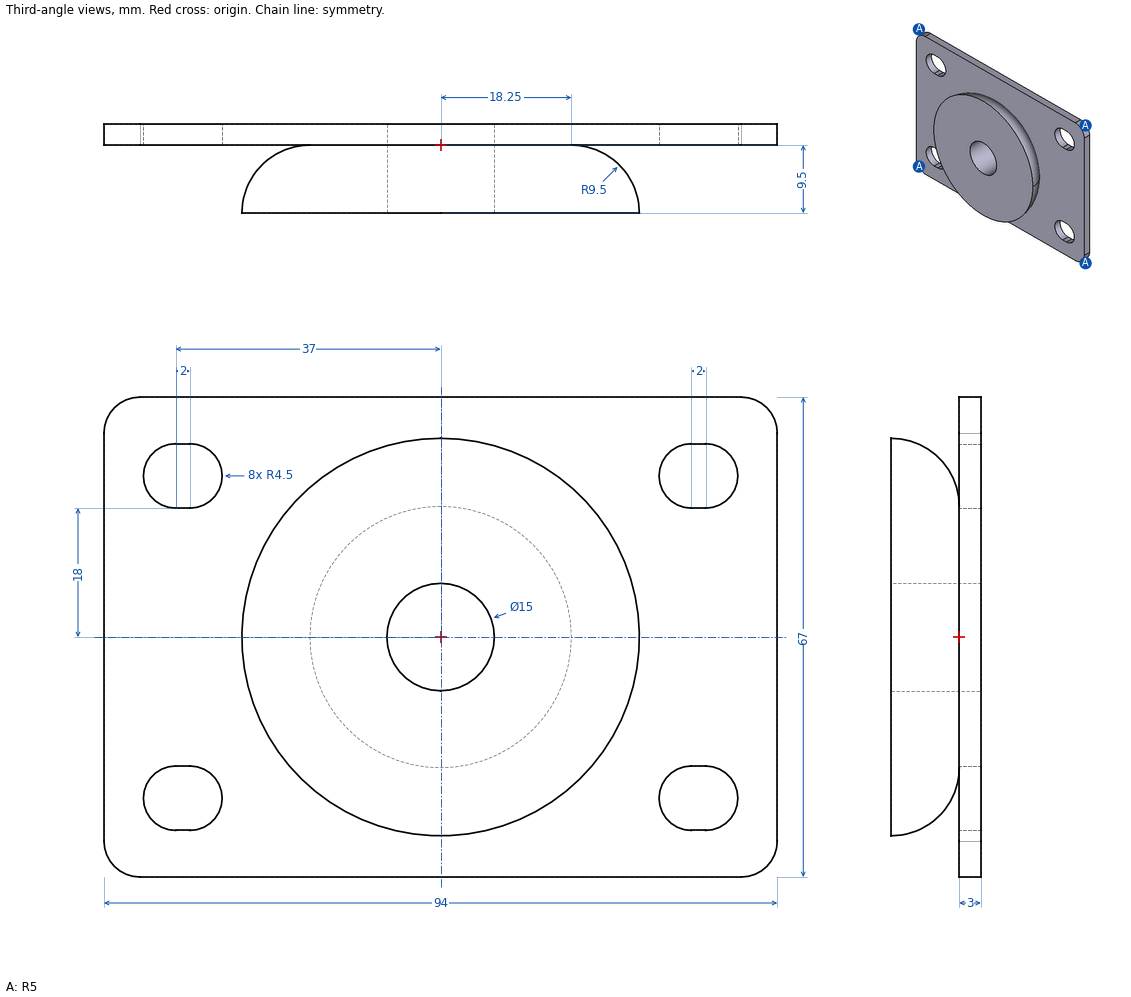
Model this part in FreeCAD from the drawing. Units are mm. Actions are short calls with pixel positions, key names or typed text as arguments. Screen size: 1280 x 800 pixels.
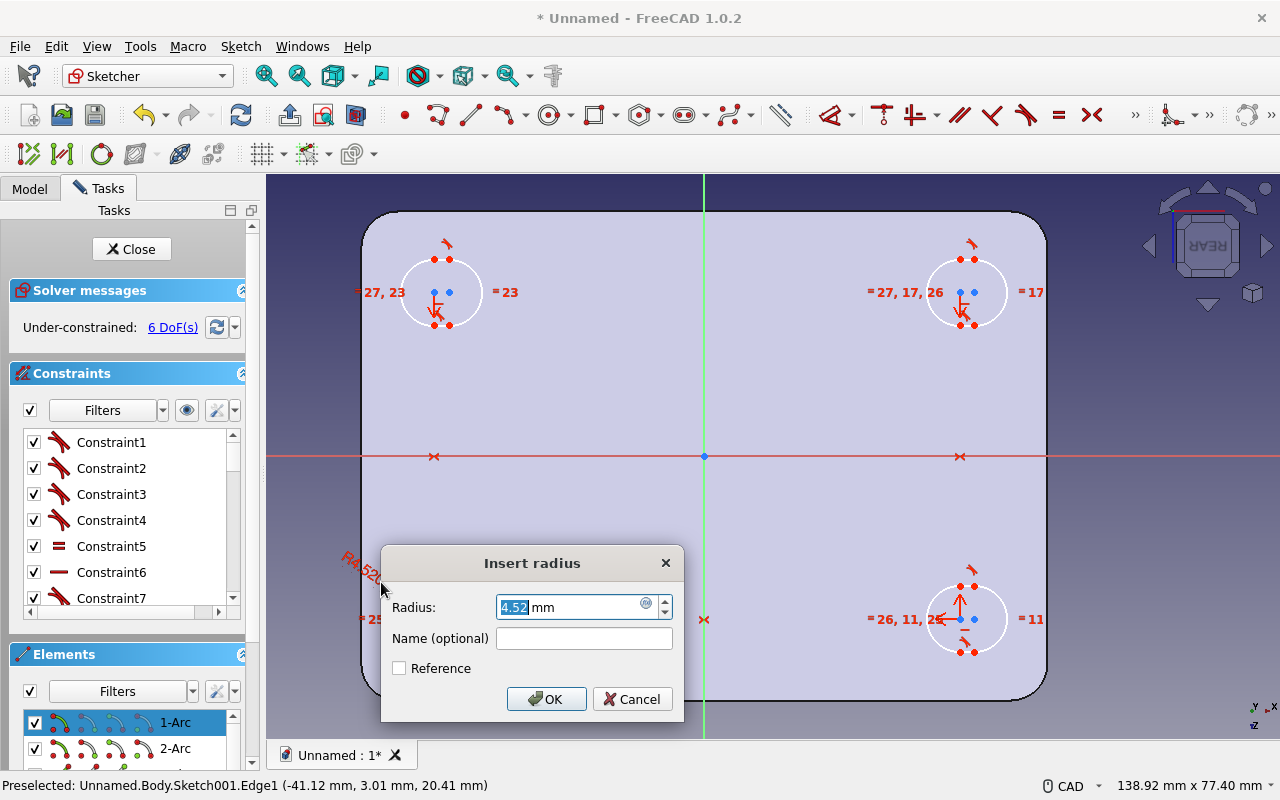
text(4.5)
key(Return)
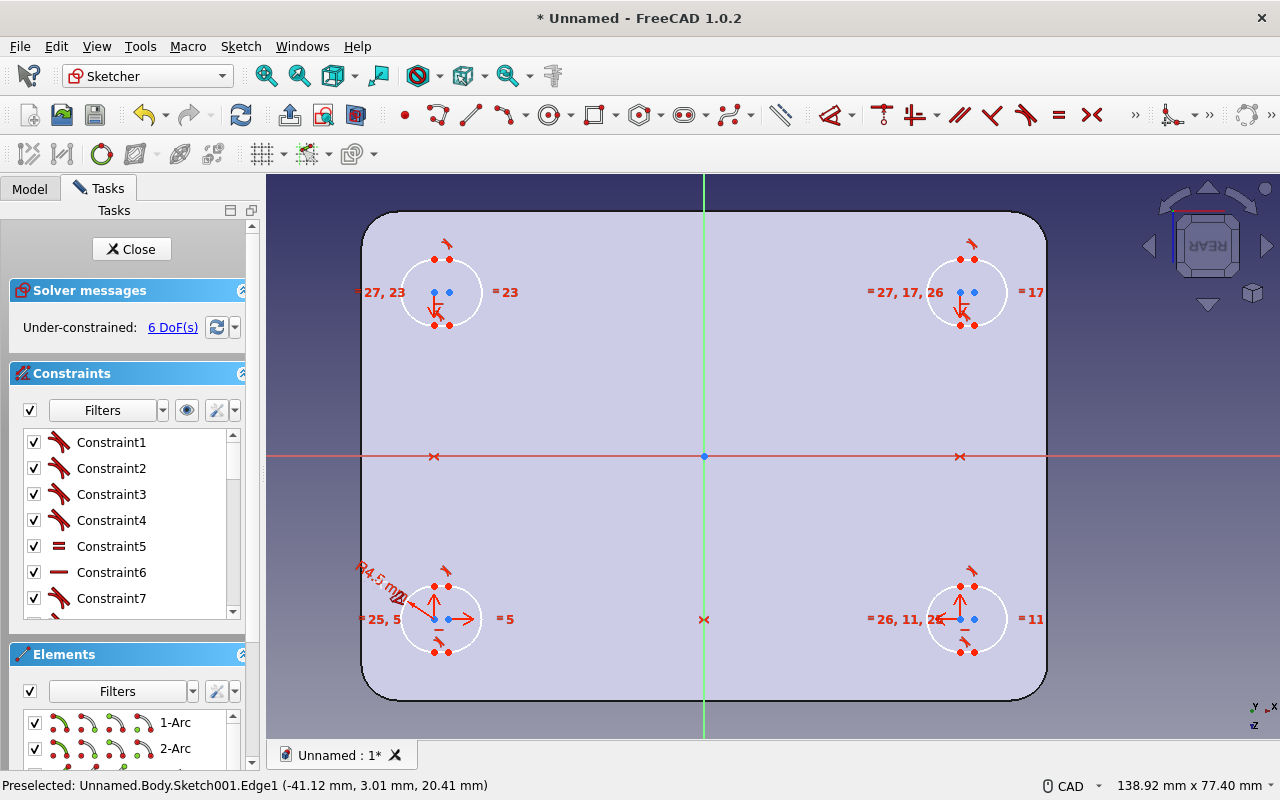
scroll(441, 586, up, 6)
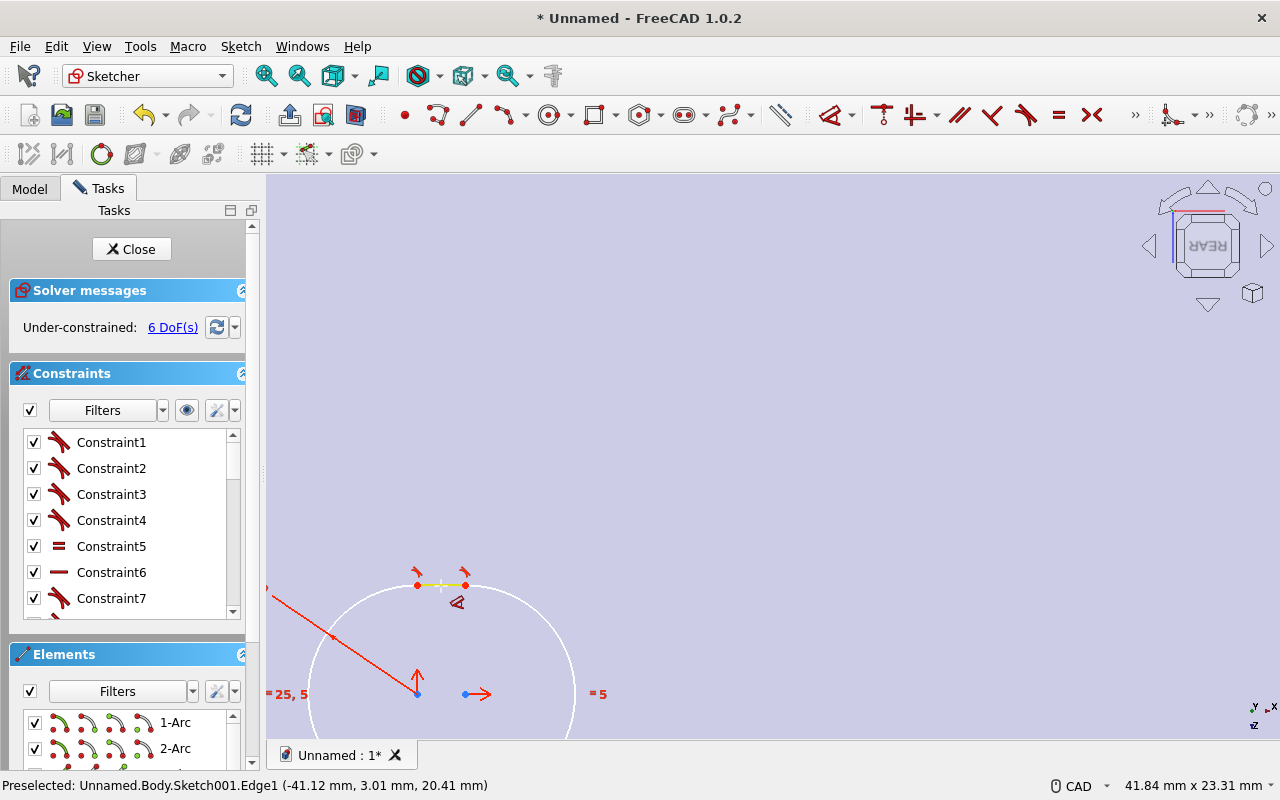
click(442, 585)
click(442, 619)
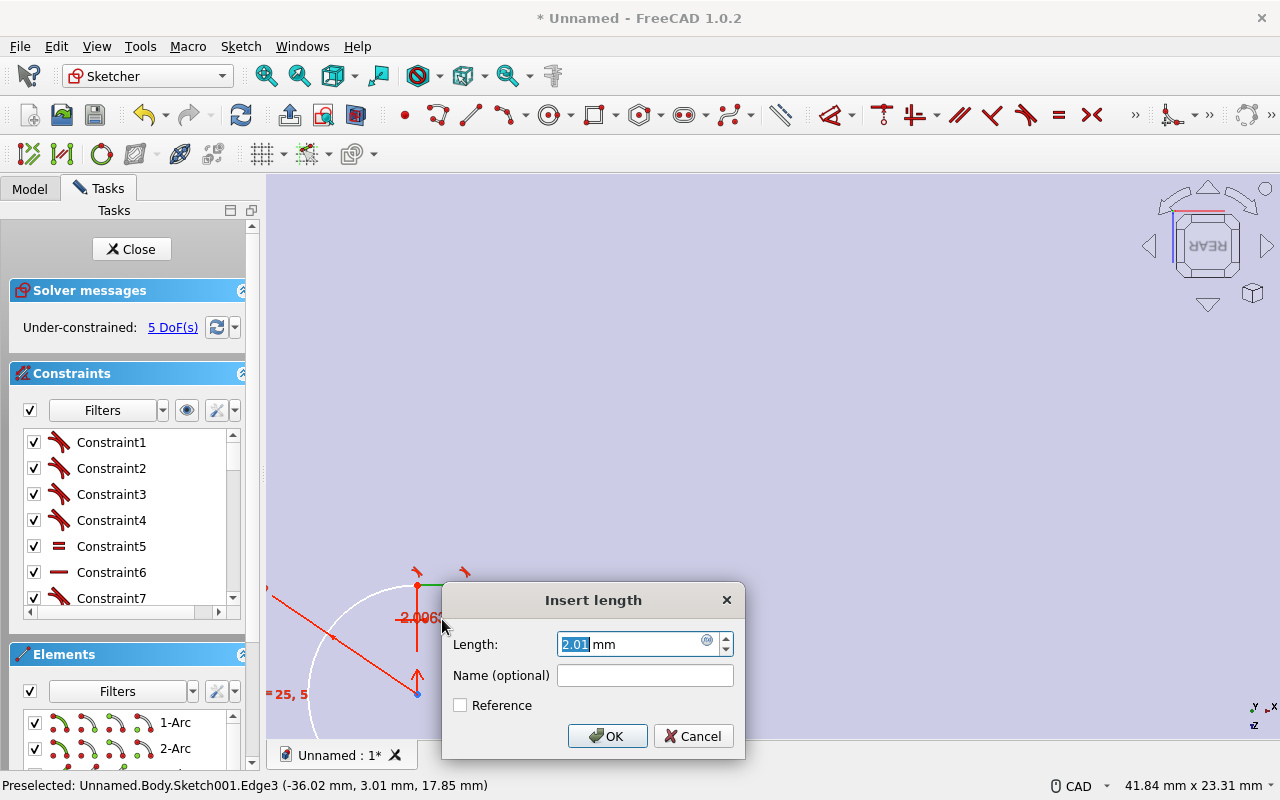
text(2)
key(Return)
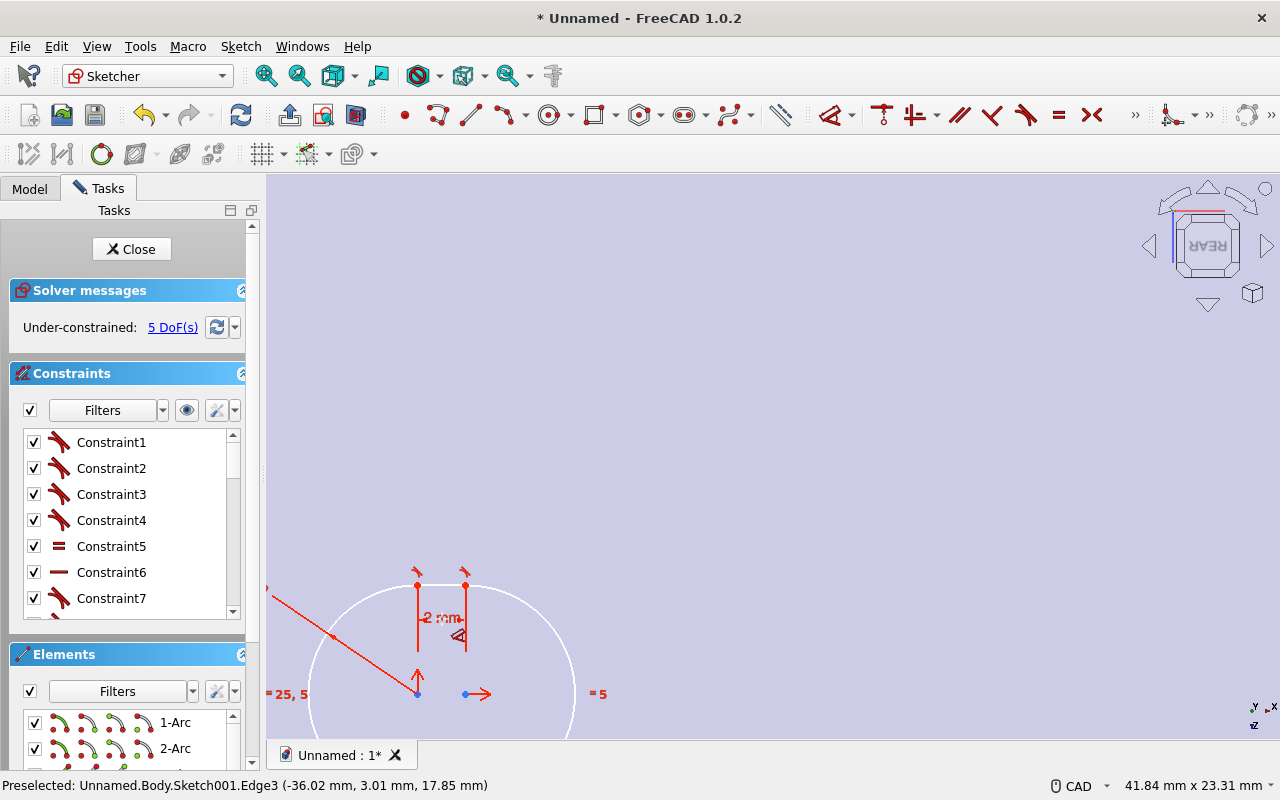
scroll(441, 587, down, 6)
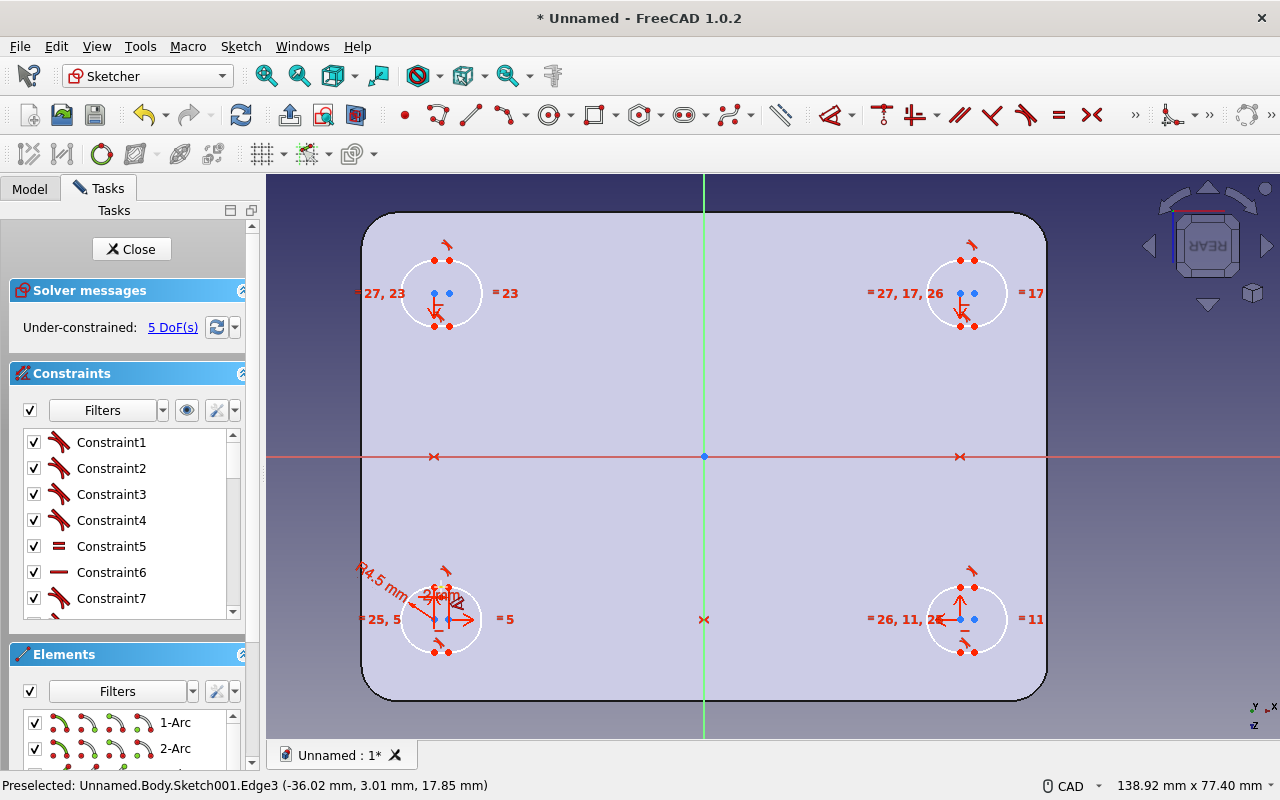
scroll(964, 587, up, 6)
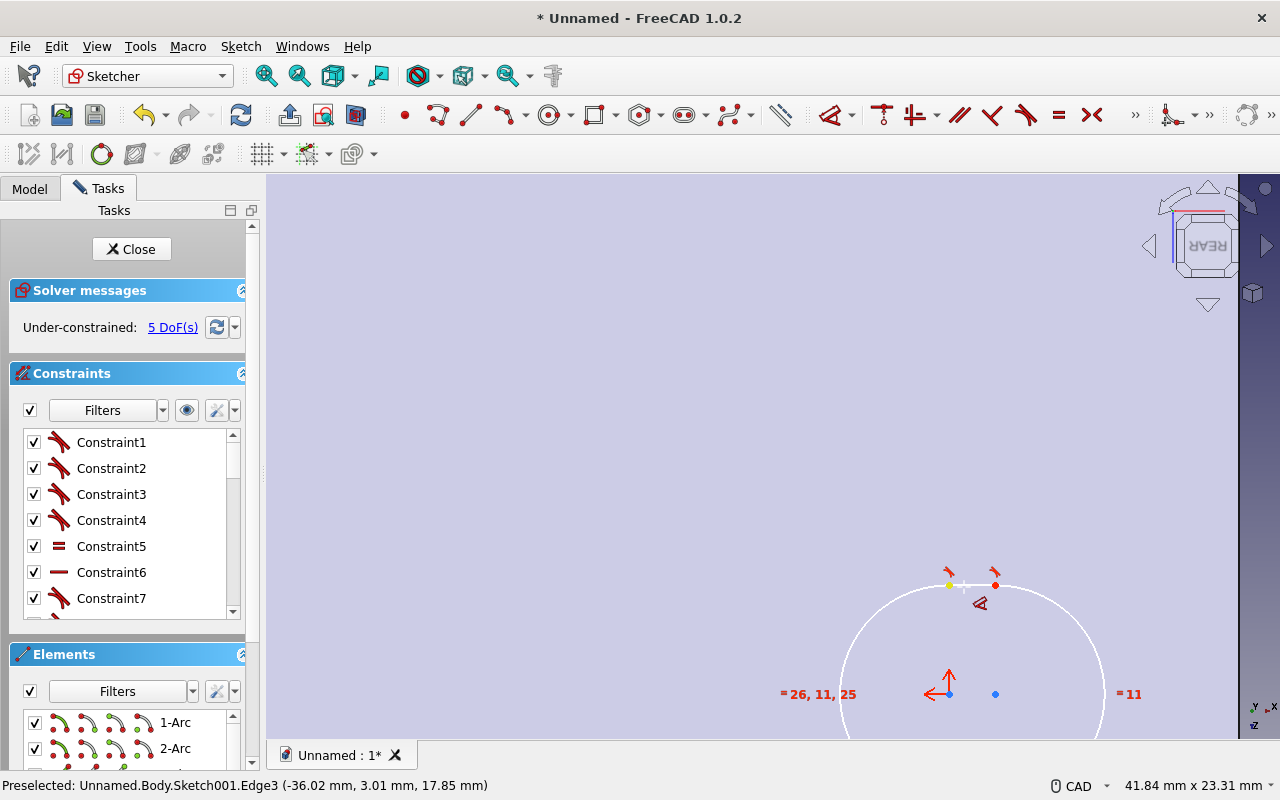
click(963, 585)
click(972, 619)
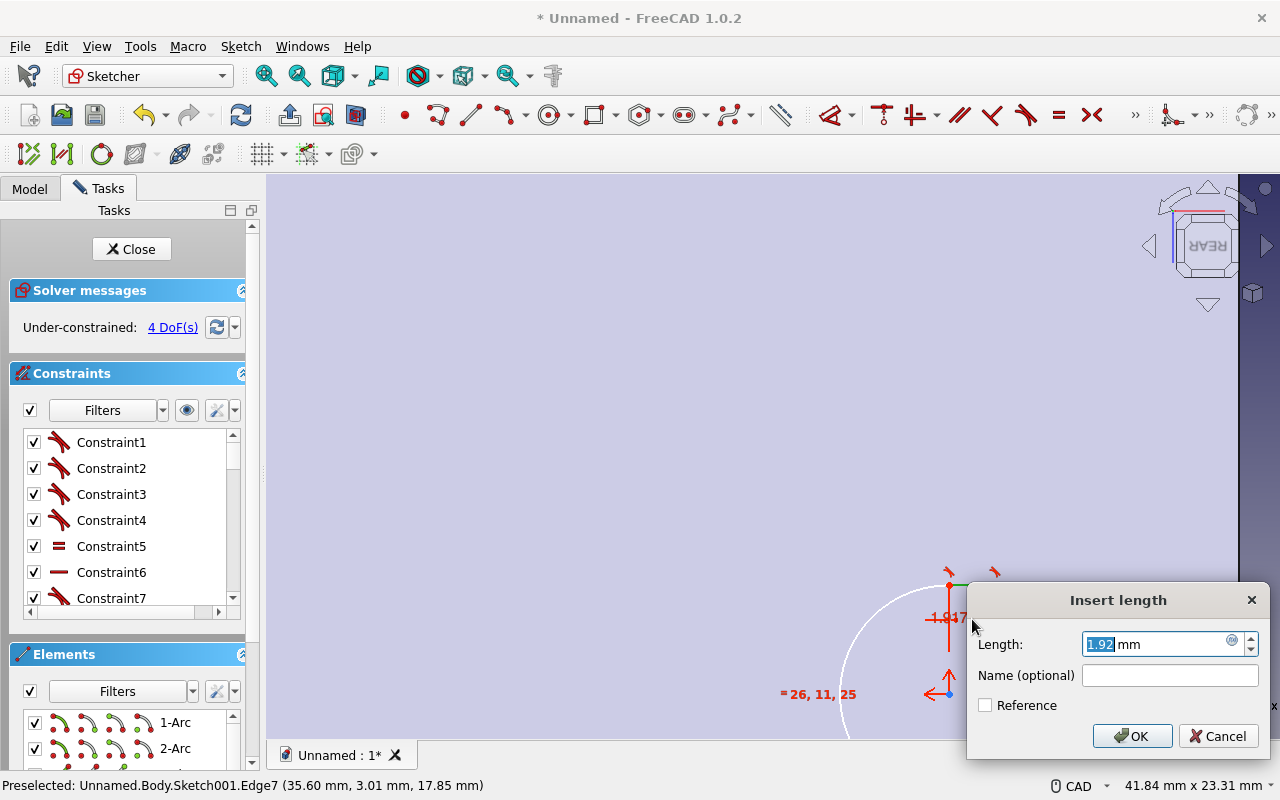
text(2)
key(Return)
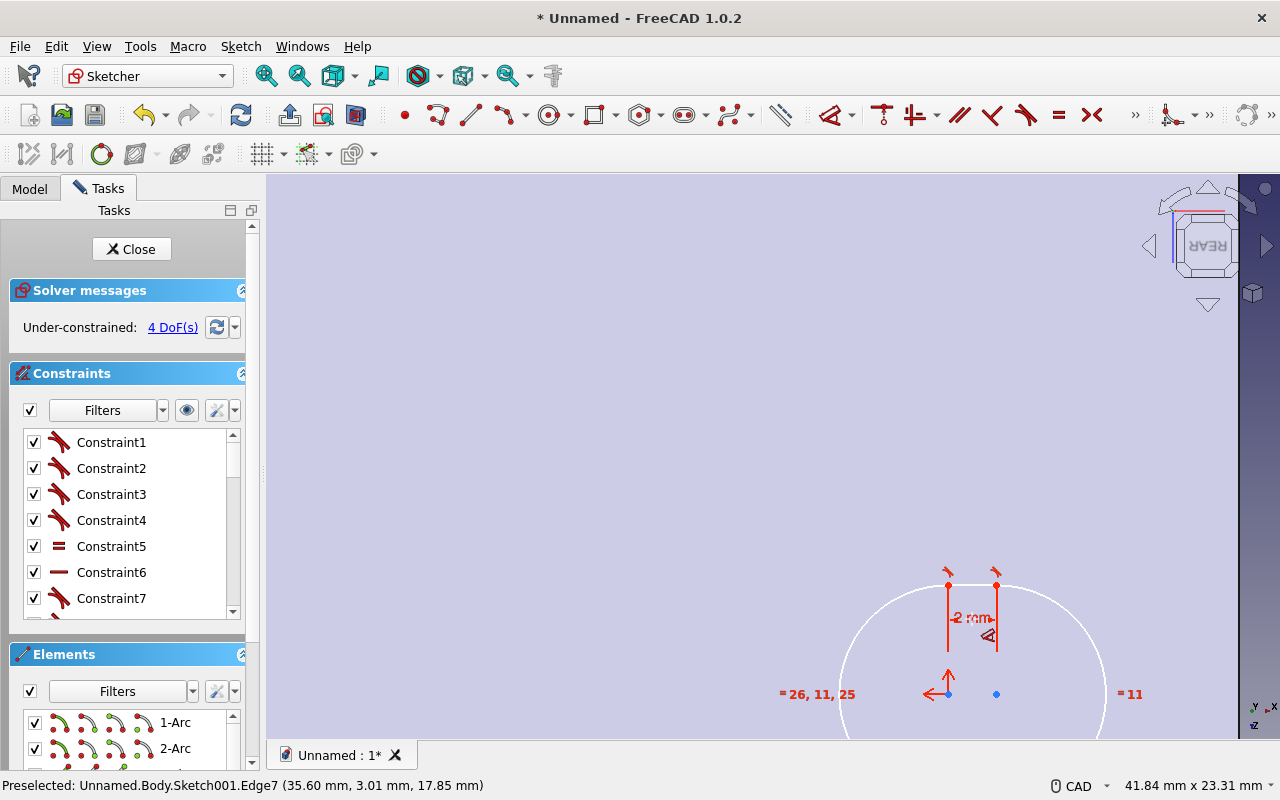
scroll(965, 587, down, 6)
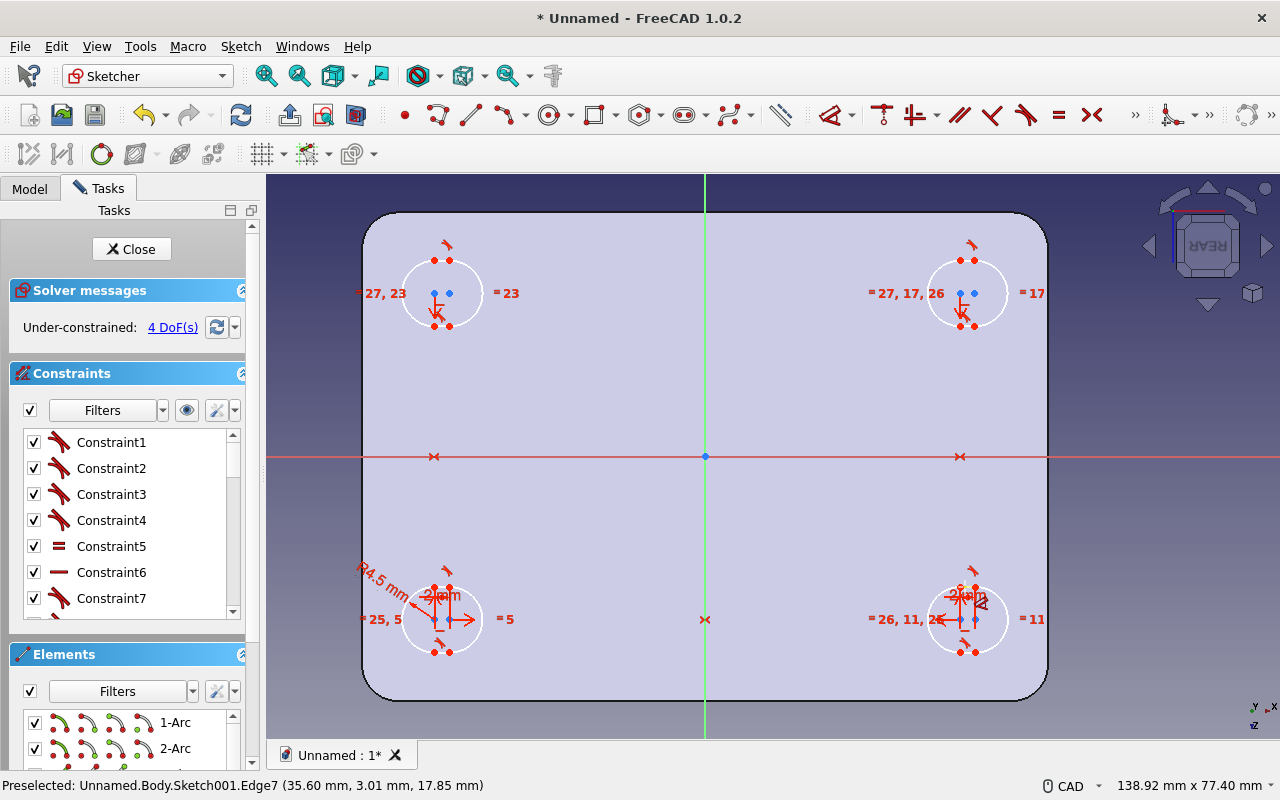
scroll(965, 261, up, 6)